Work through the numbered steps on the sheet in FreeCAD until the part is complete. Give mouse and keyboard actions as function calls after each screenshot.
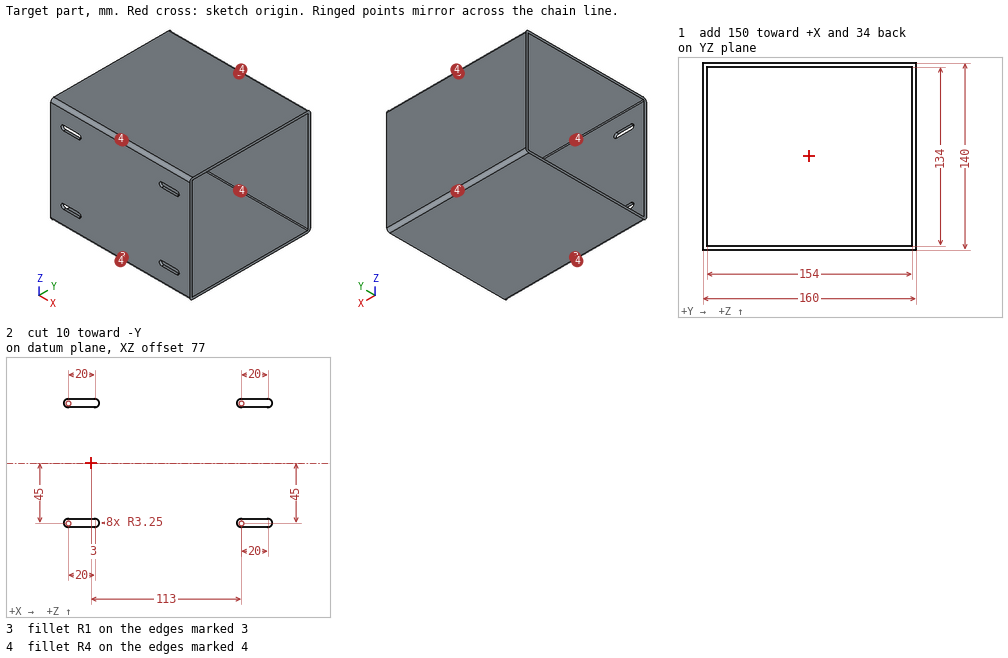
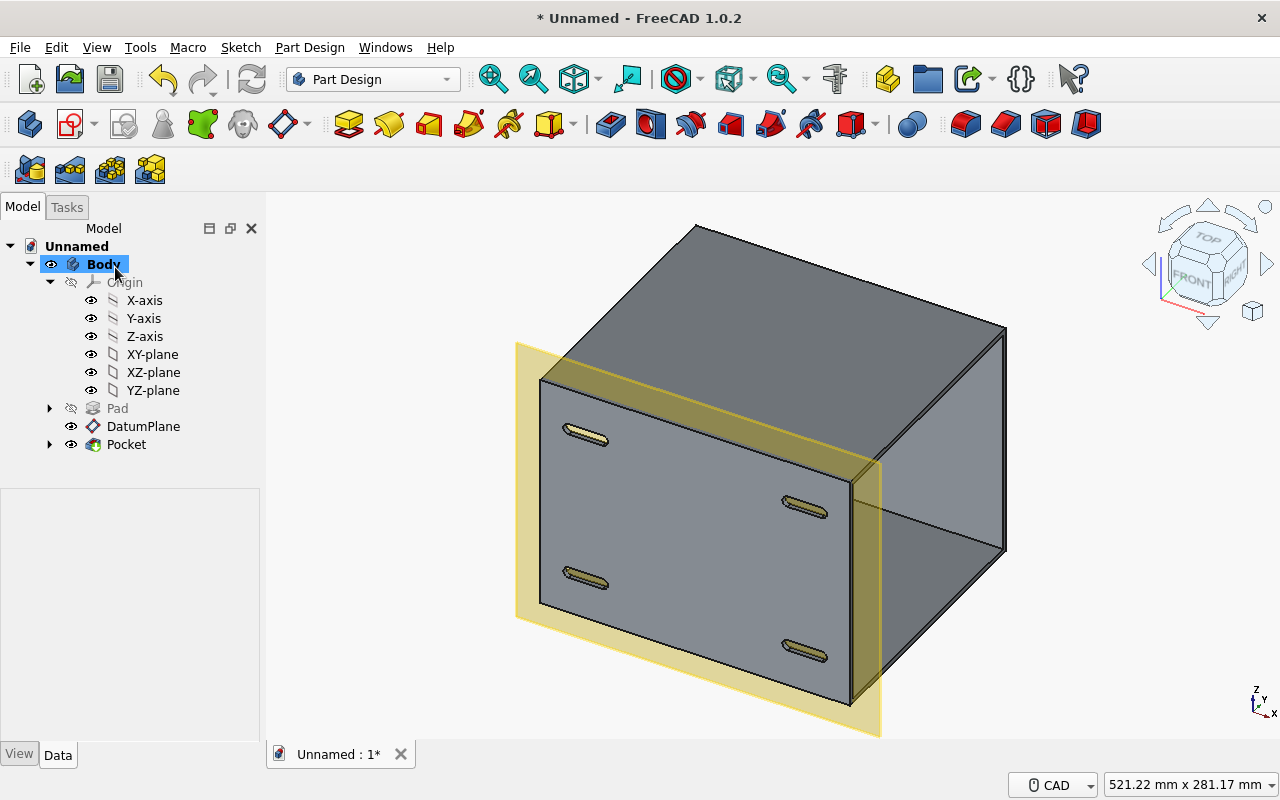
click(116, 426)
key(space)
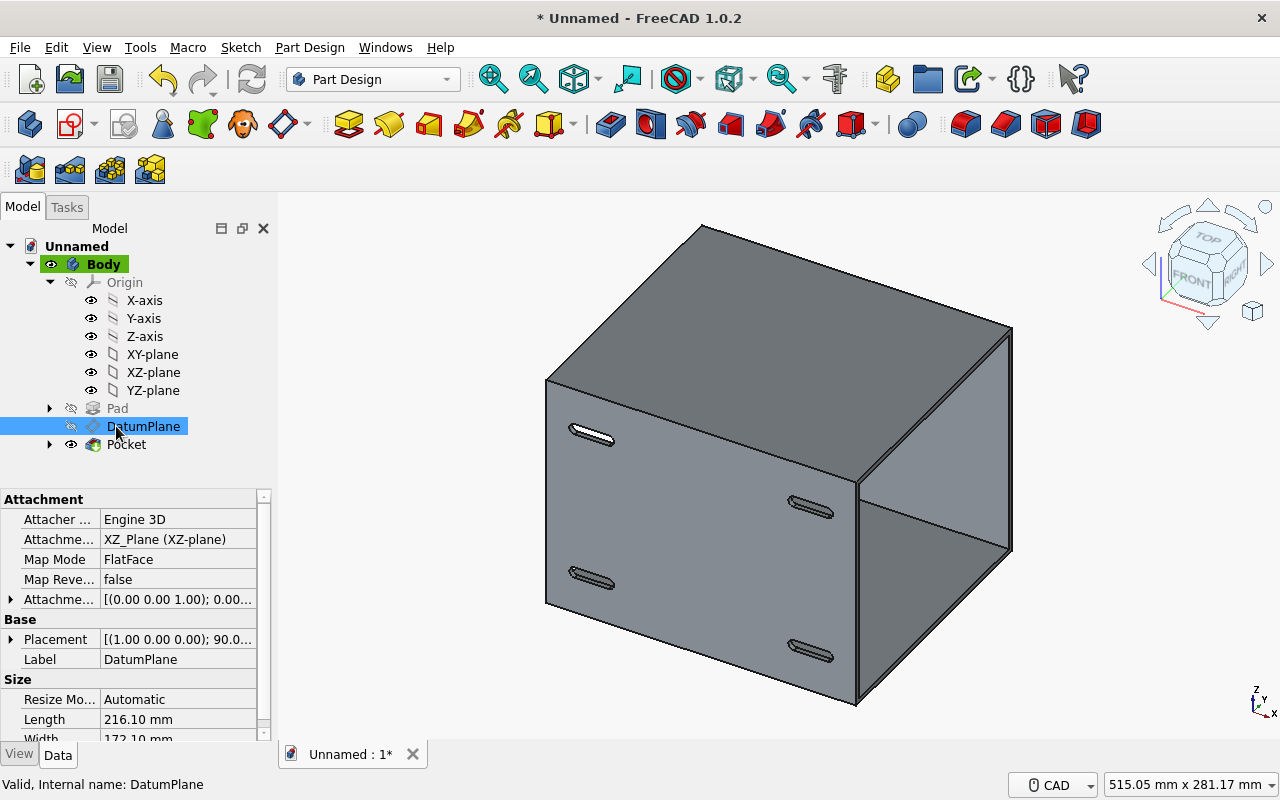
key(0)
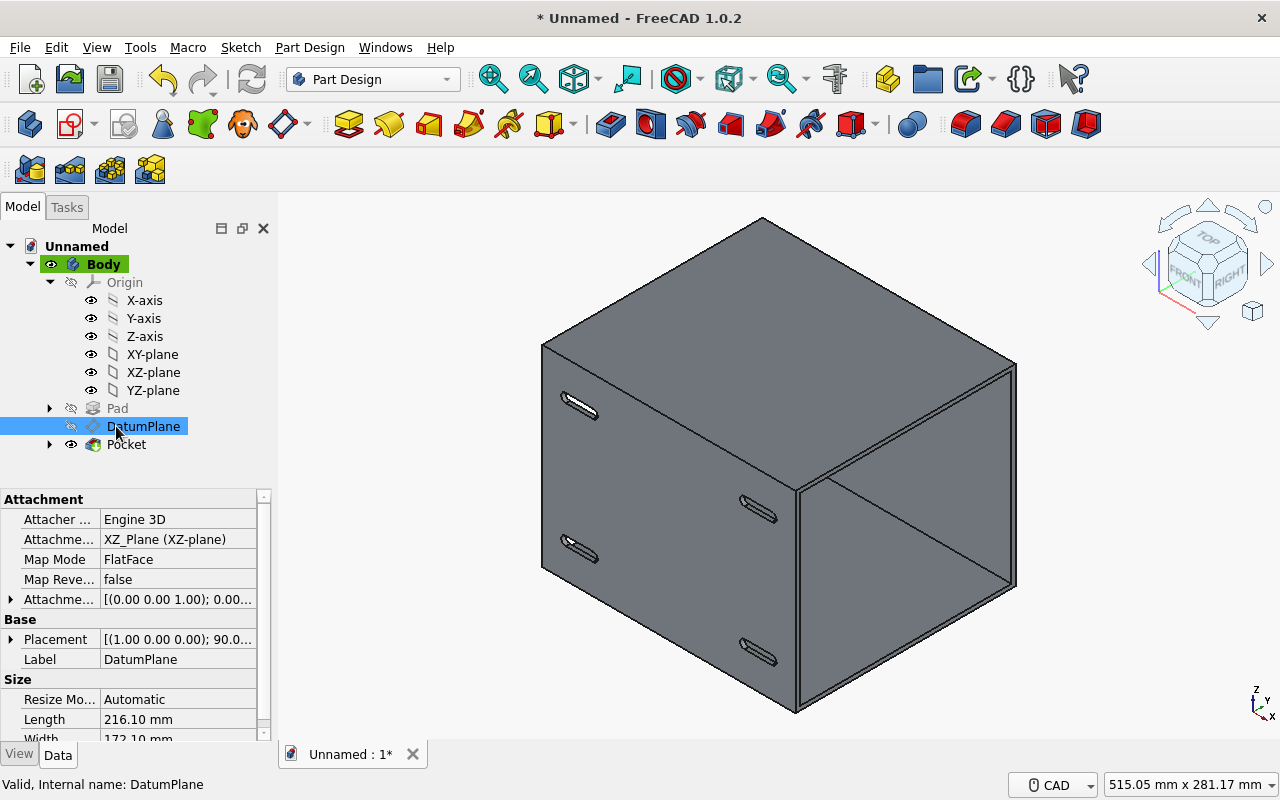
key(2)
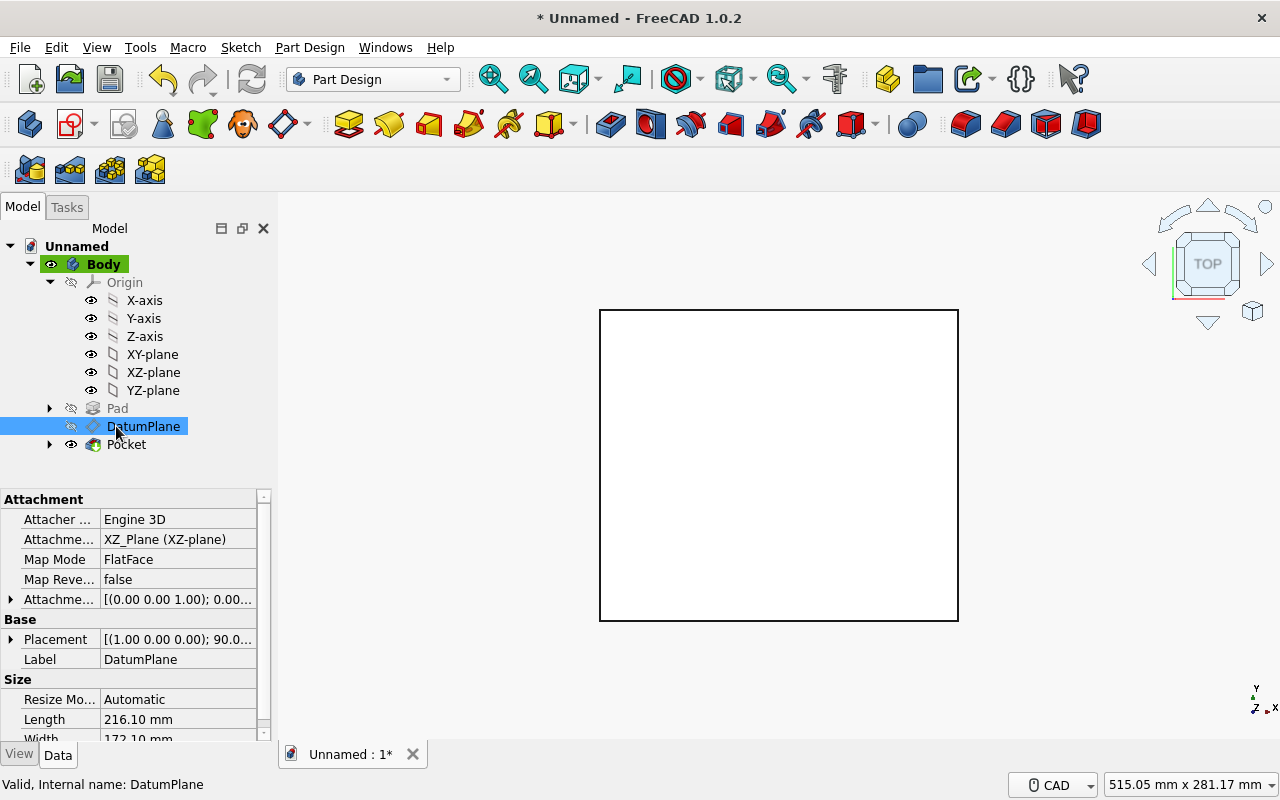
key(1)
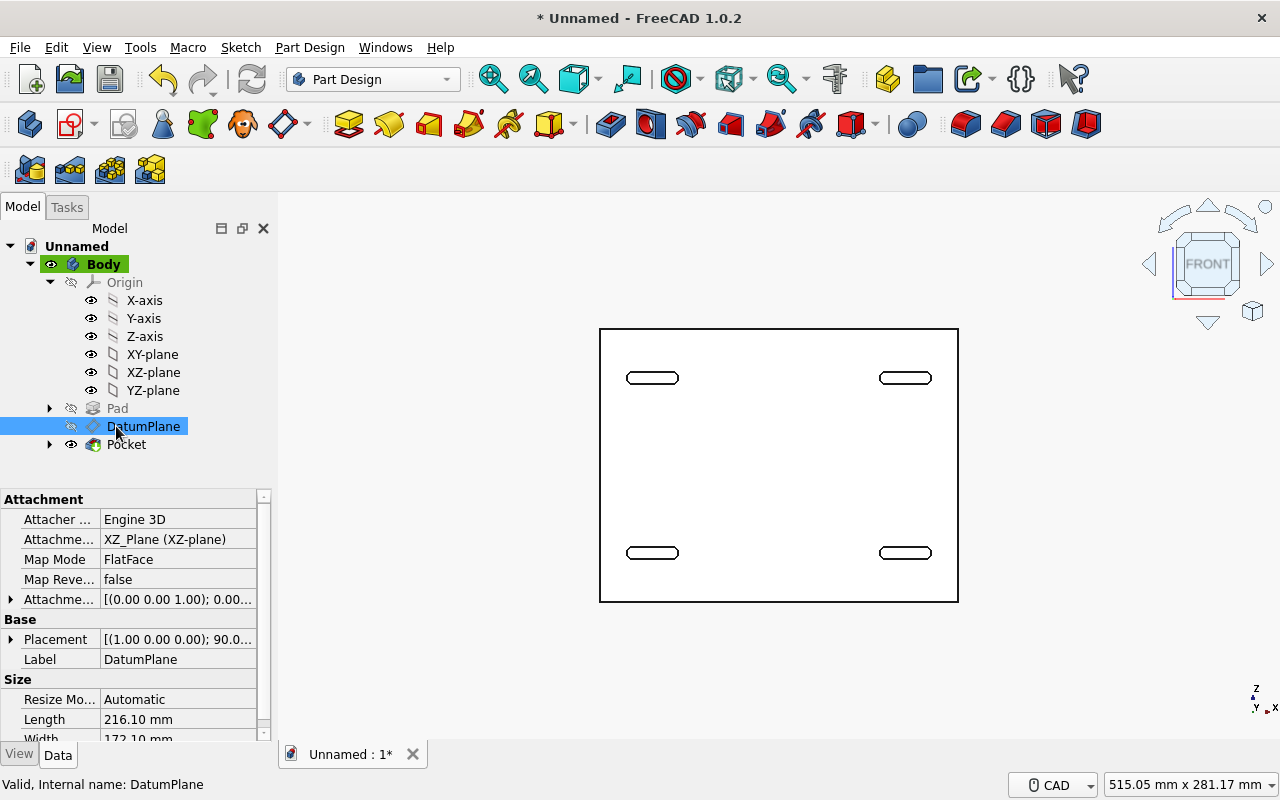
key(3)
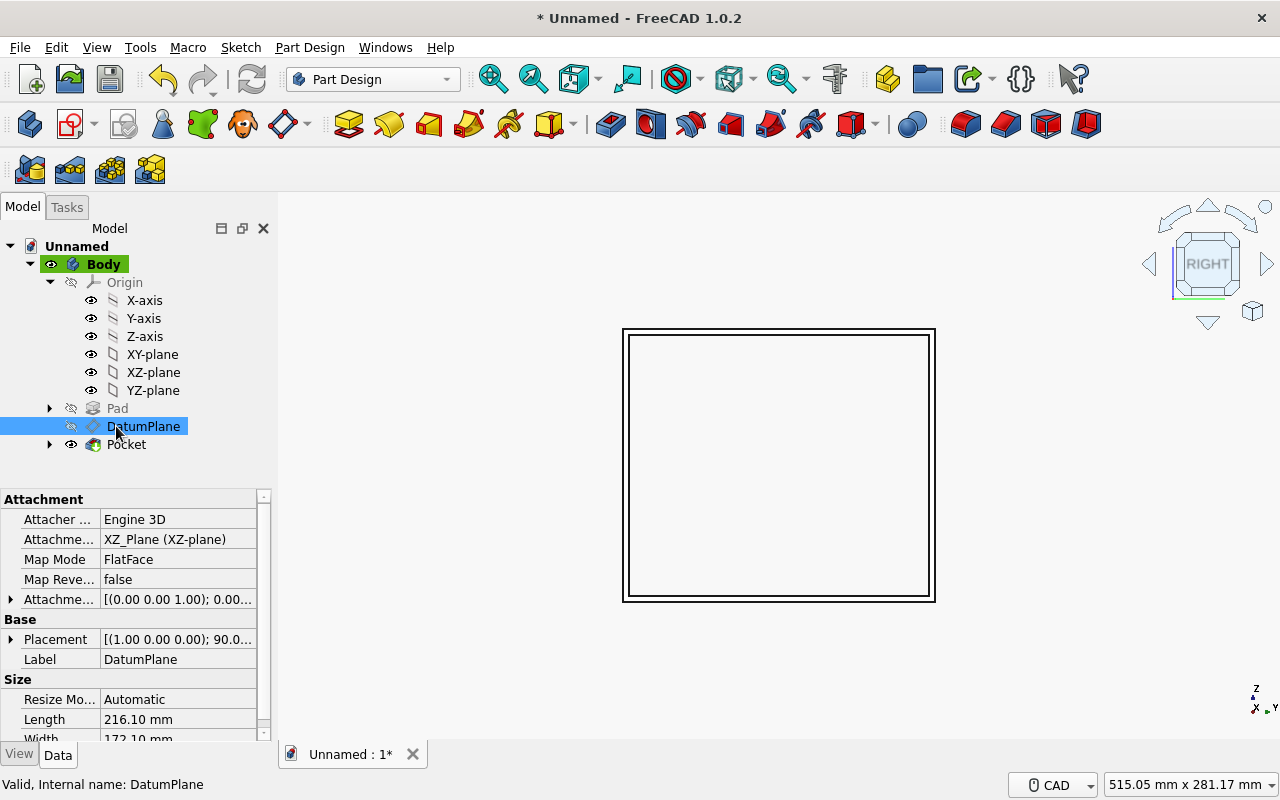
key(5)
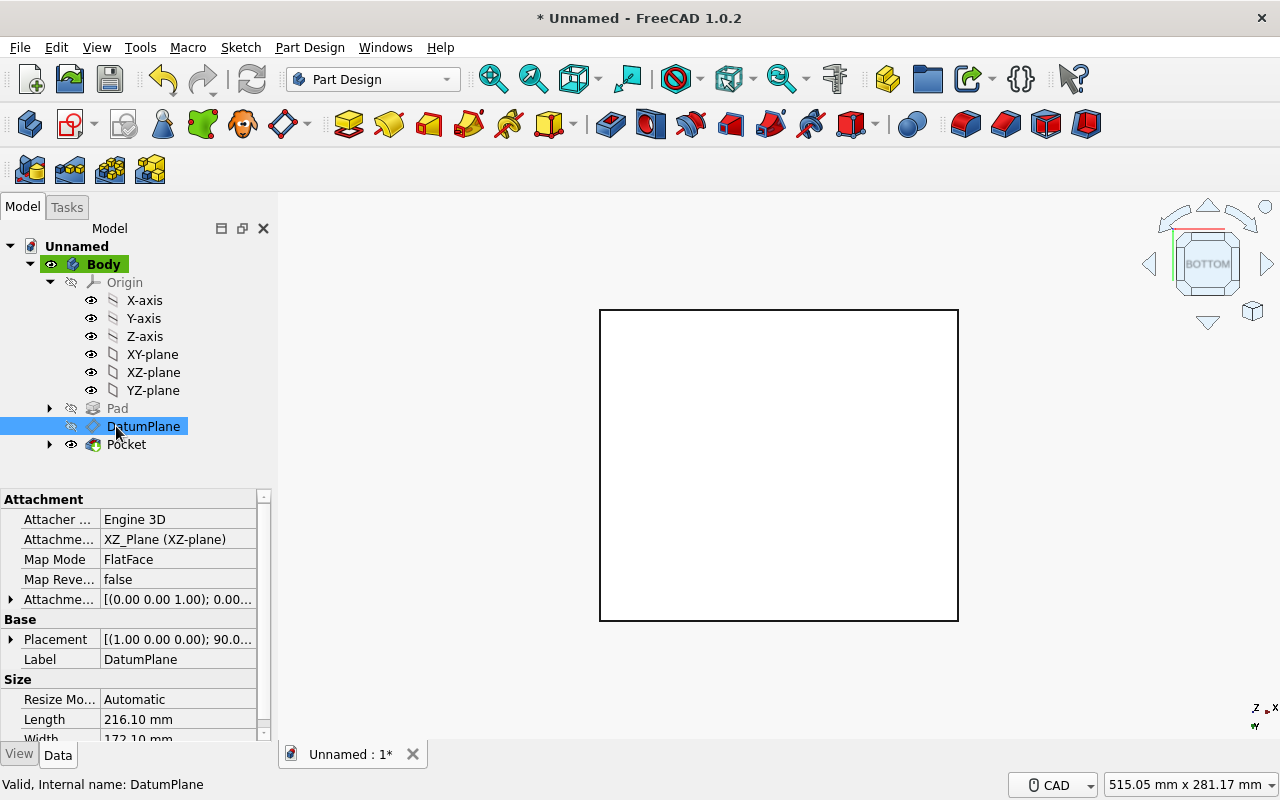
key(4)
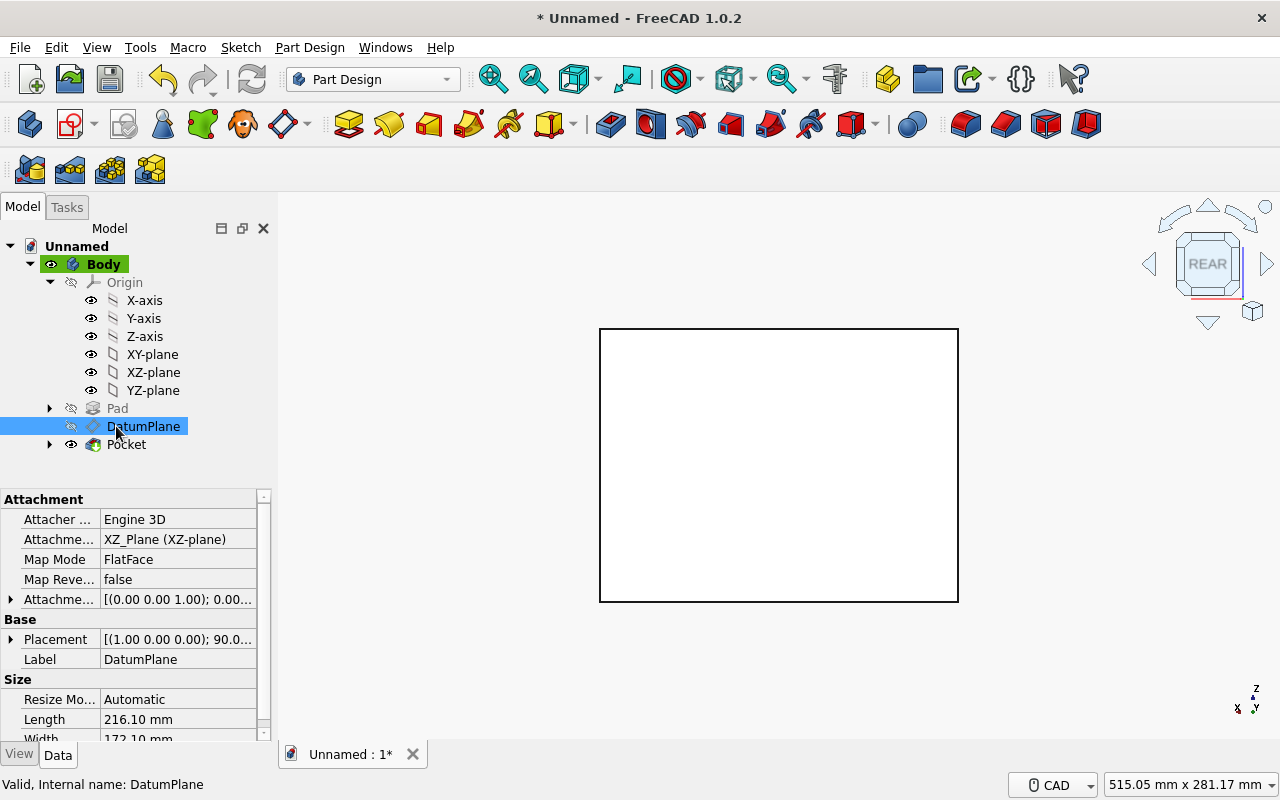
key(6)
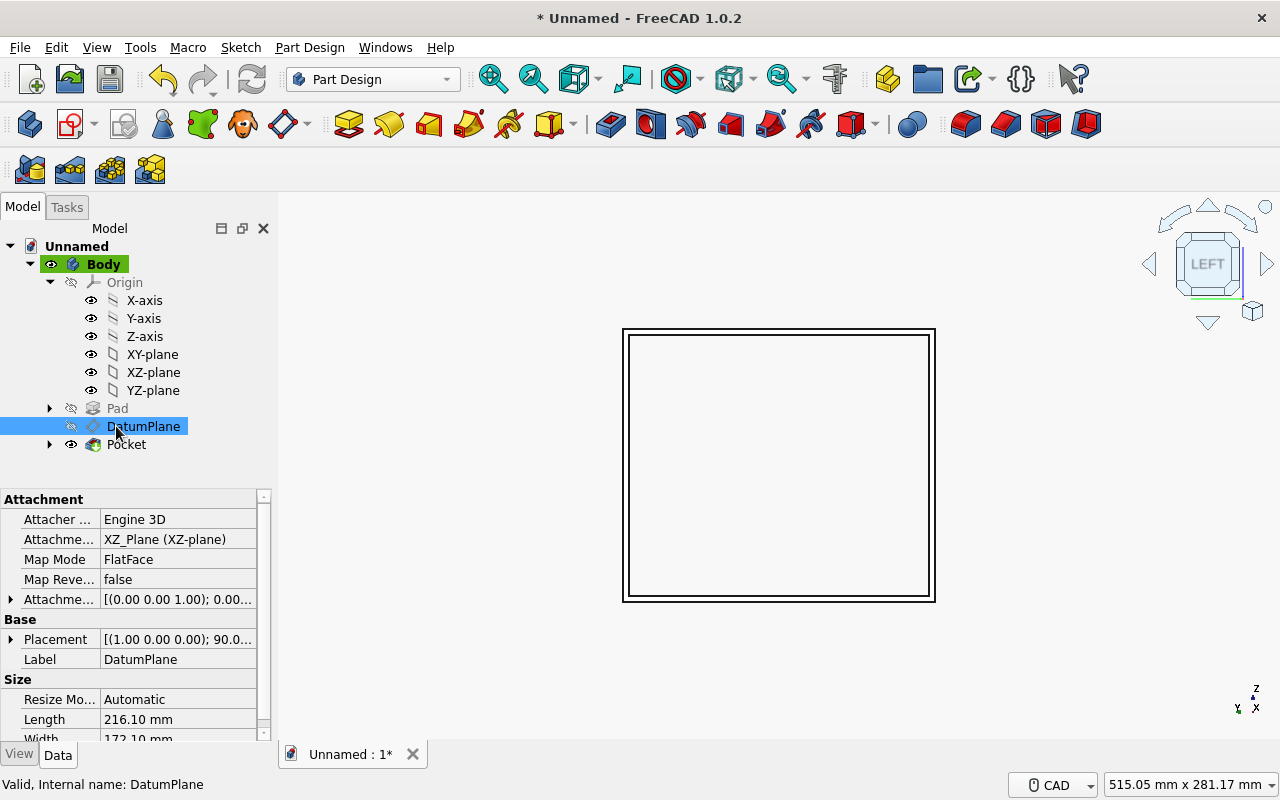
key(v)
key(3)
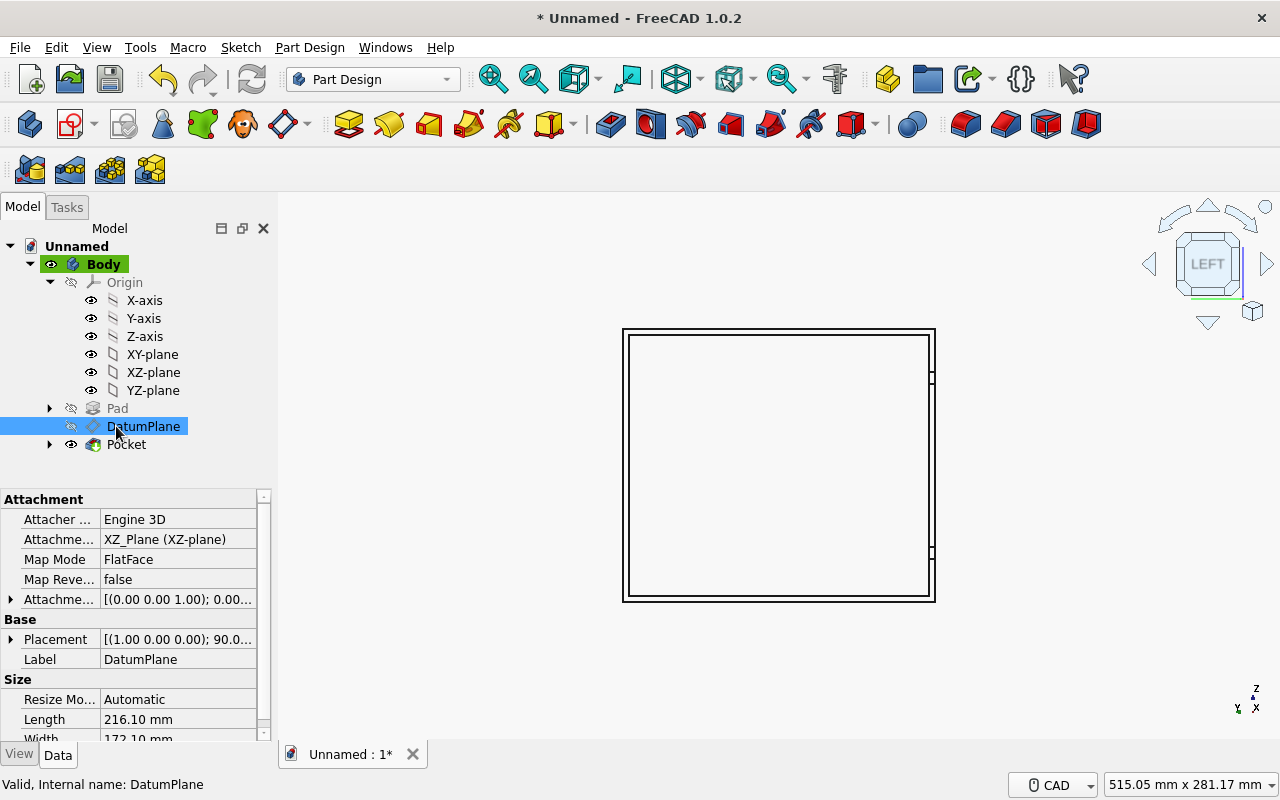
key(0)